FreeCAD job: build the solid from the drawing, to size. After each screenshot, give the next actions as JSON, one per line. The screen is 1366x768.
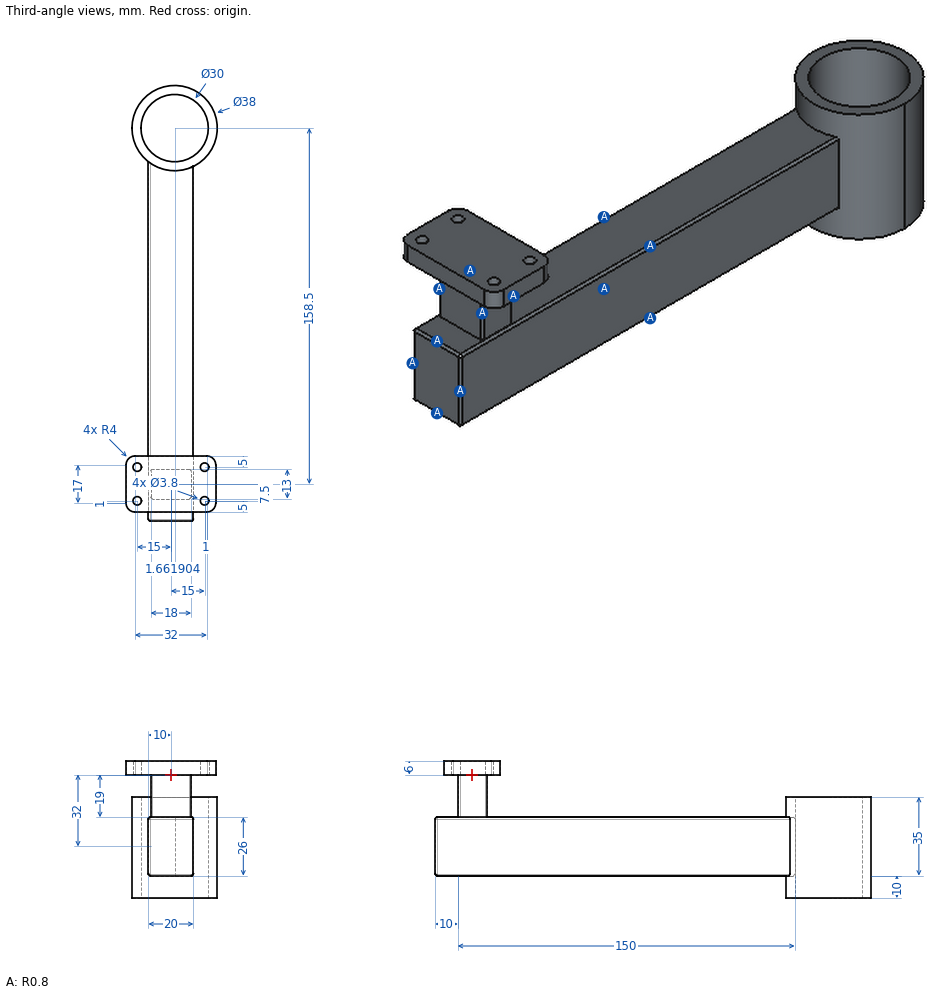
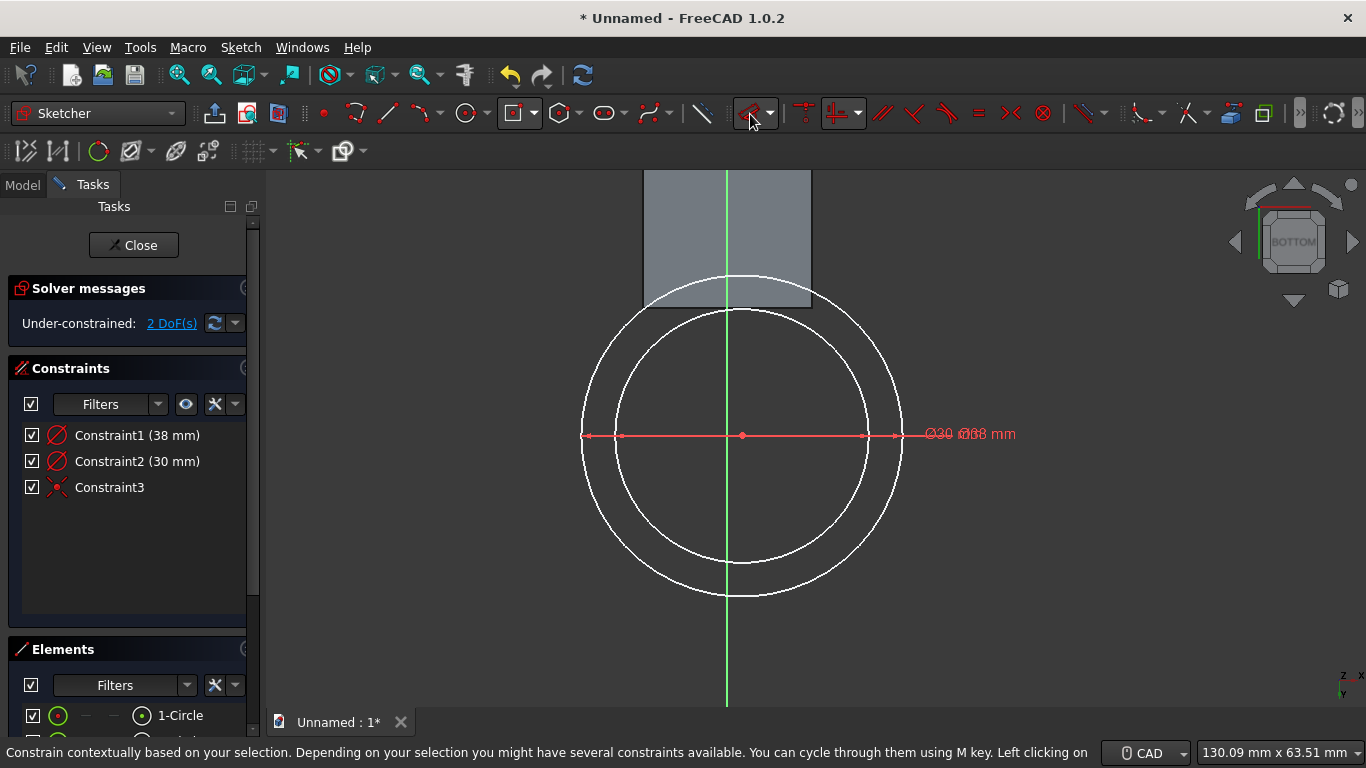
{"action": "left_click", "coordinate": [742, 436]}
{"action": "left_click", "coordinate": [693, 262]}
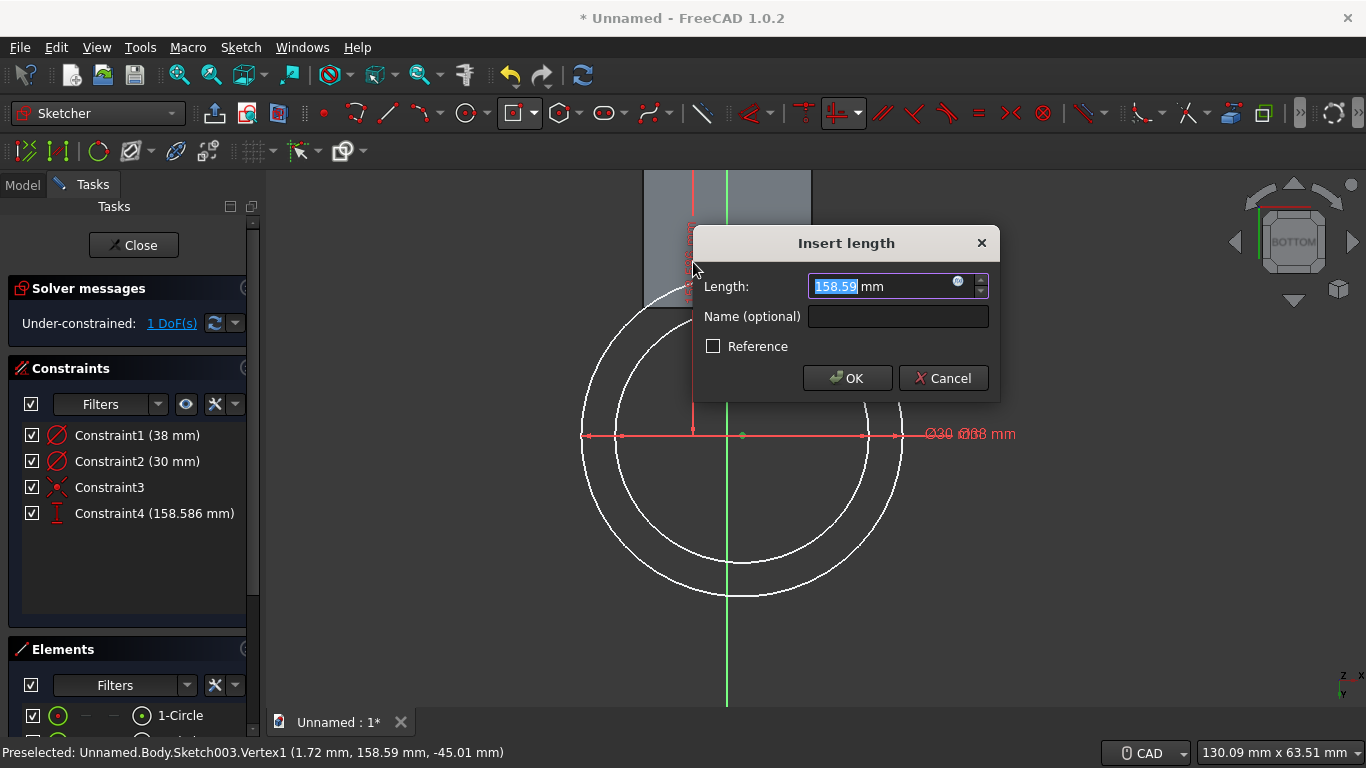
{"action": "type", "text": "158.5"}
{"action": "key", "text": "Return"}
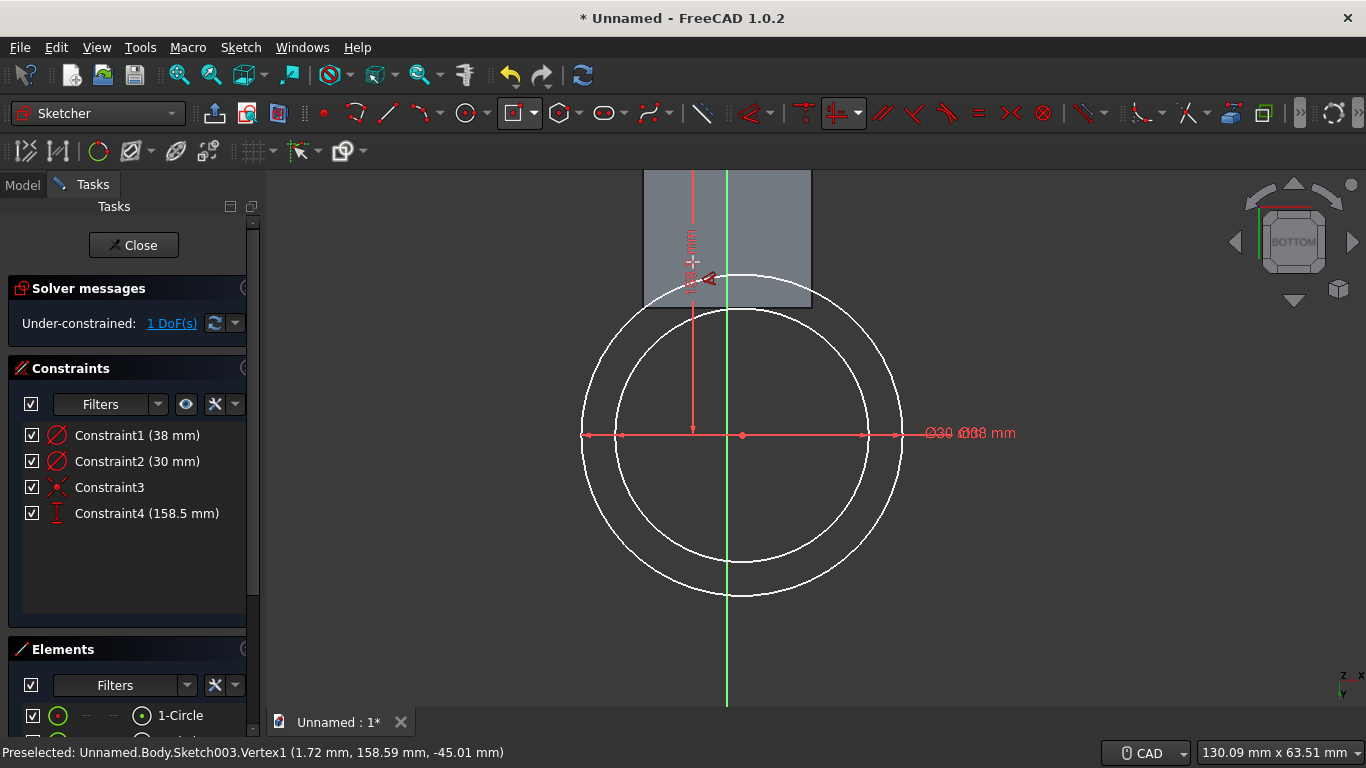
{"action": "scroll", "coordinate": [742, 435], "scroll_direction": "up", "scroll_amount": 6}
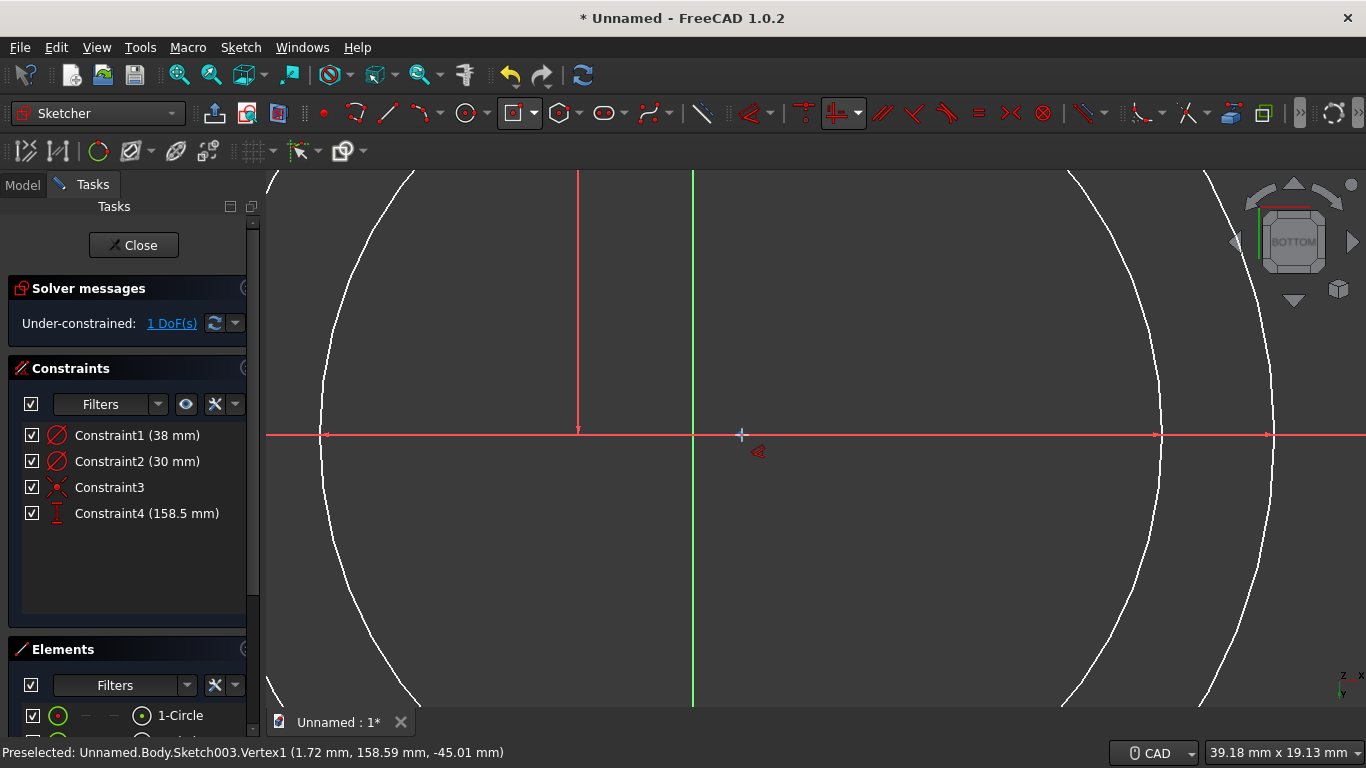
{"action": "left_click", "coordinate": [741, 435]}
{"action": "left_click", "coordinate": [717, 469]}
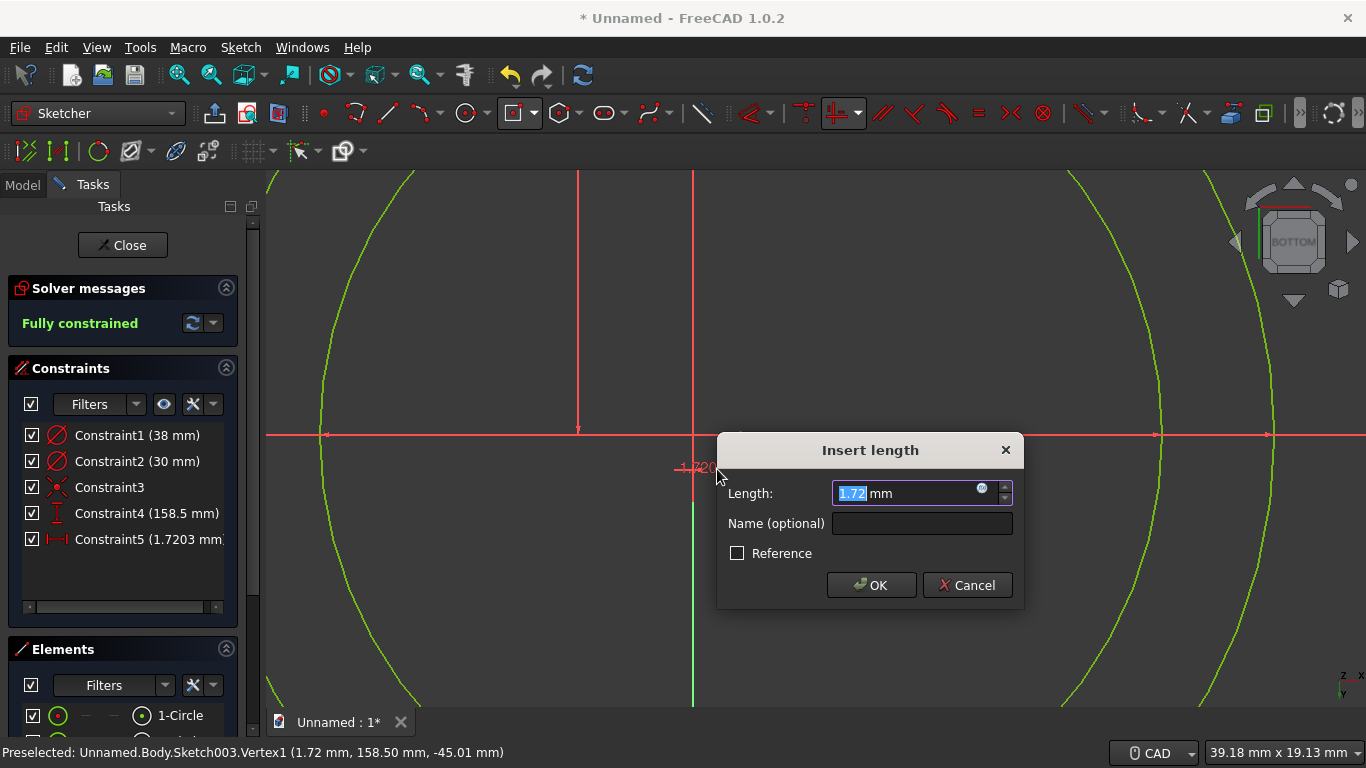
{"action": "type", "text": "1.661904"}
{"action": "key", "text": "Return"}
{"action": "key", "text": "Escape"}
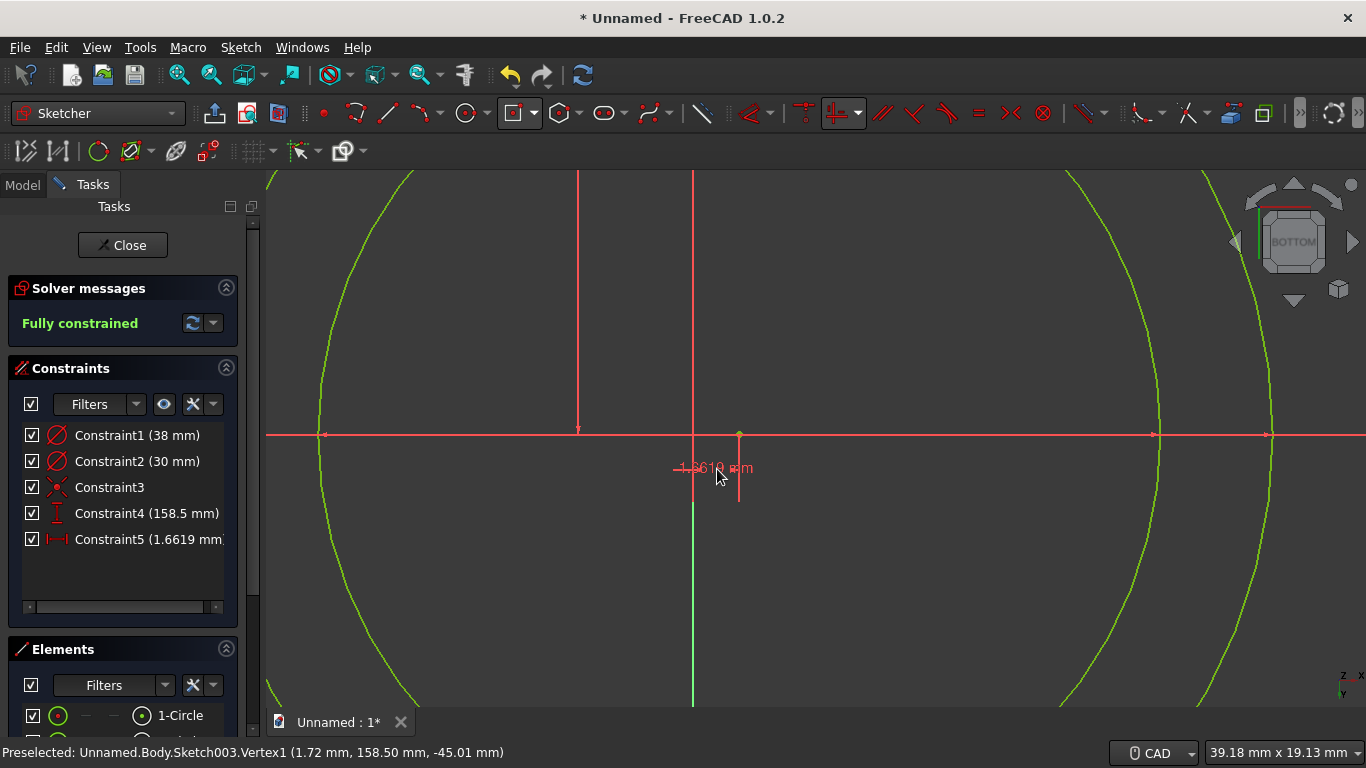
{"action": "left_click", "coordinate": [123, 245]}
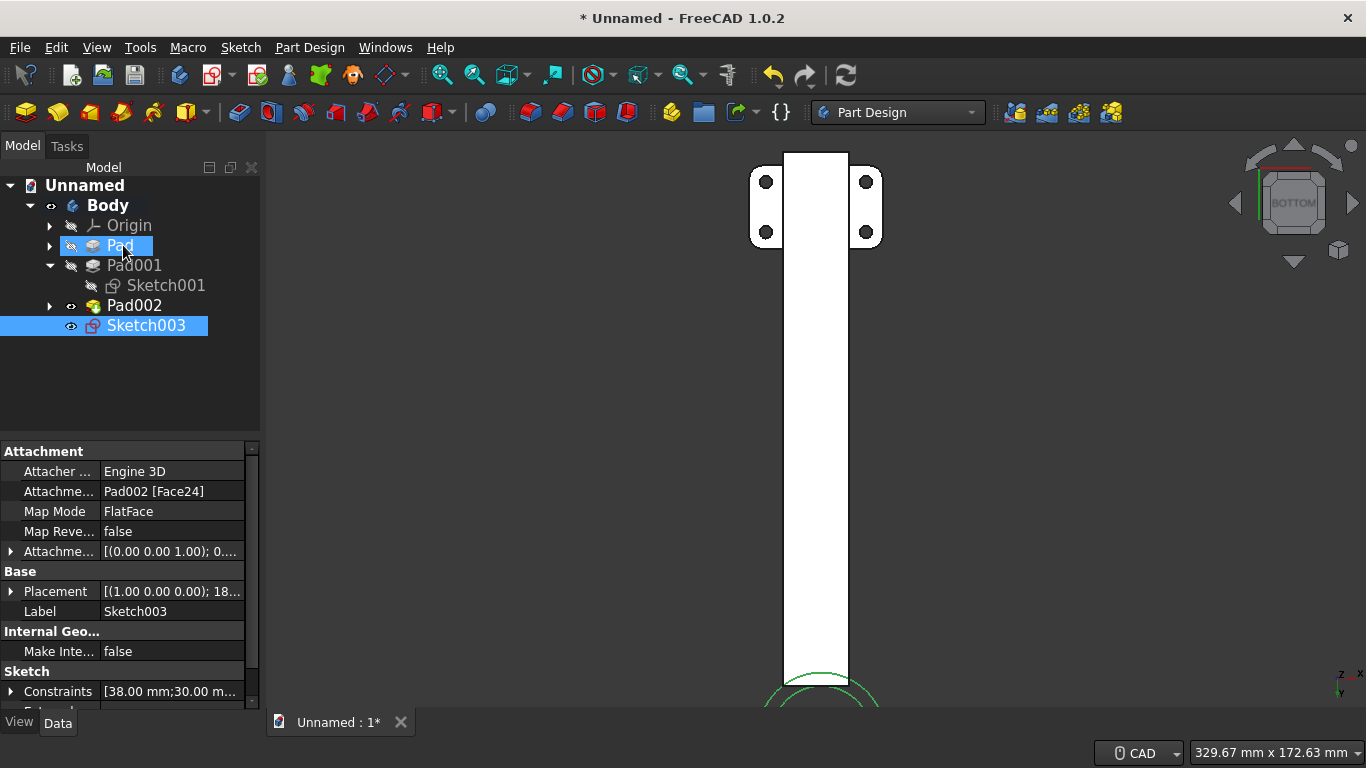
{"action": "left_click", "coordinate": [26, 112]}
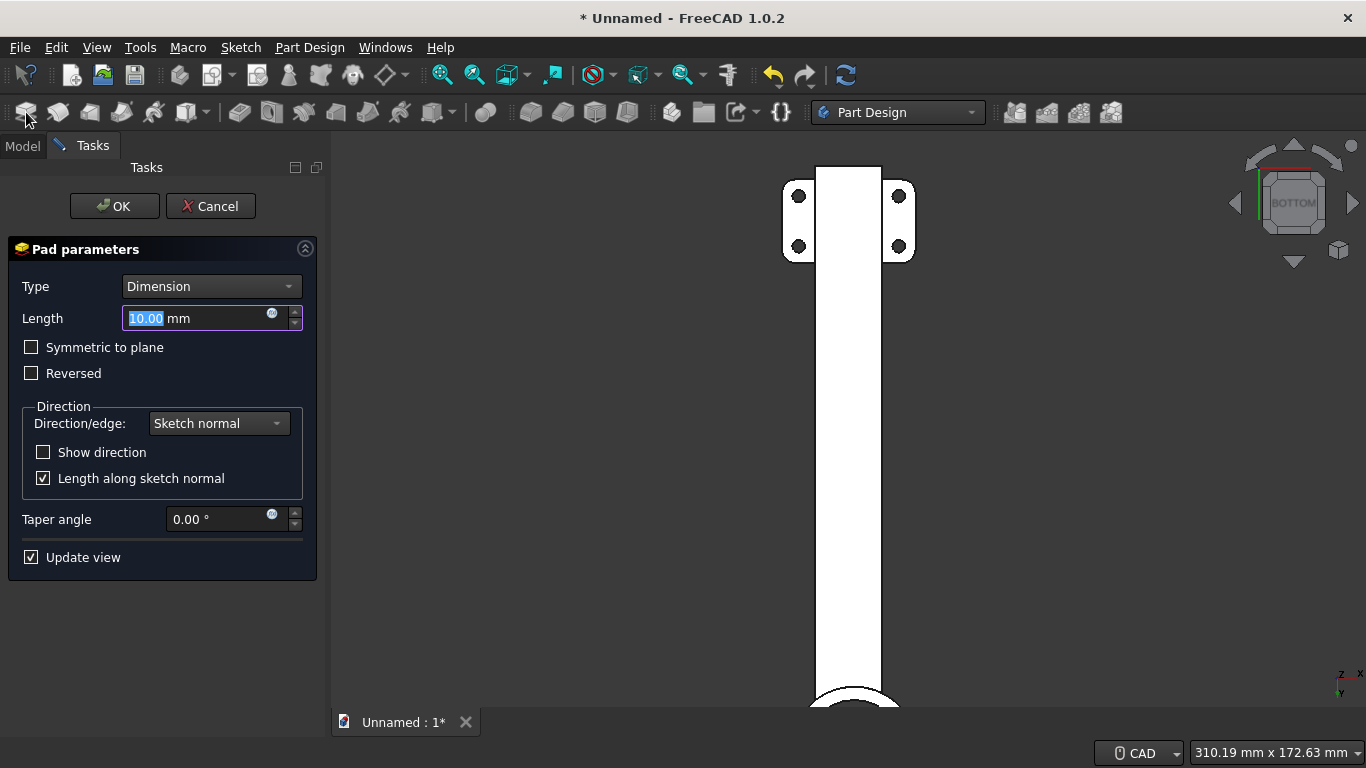
{"action": "left_click", "coordinate": [212, 286]}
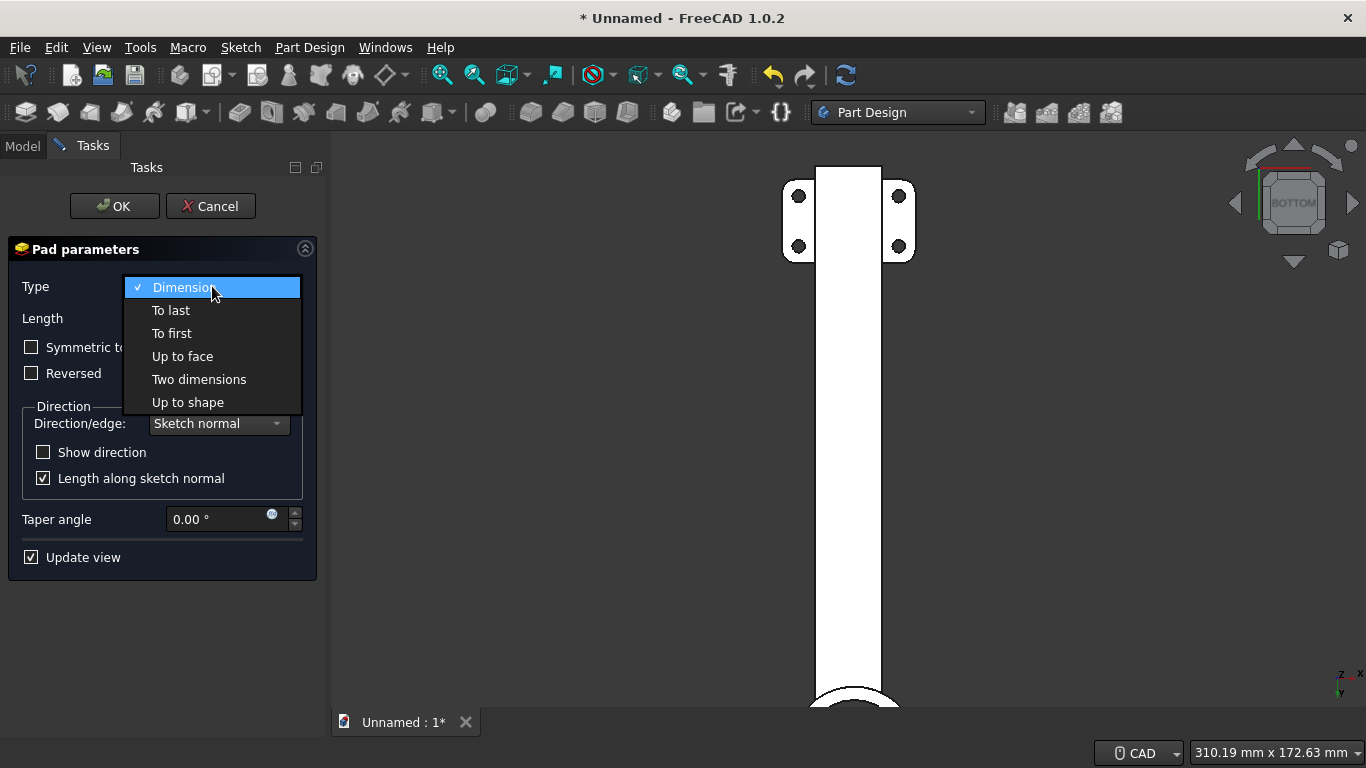
{"action": "left_click", "coordinate": [212, 380]}